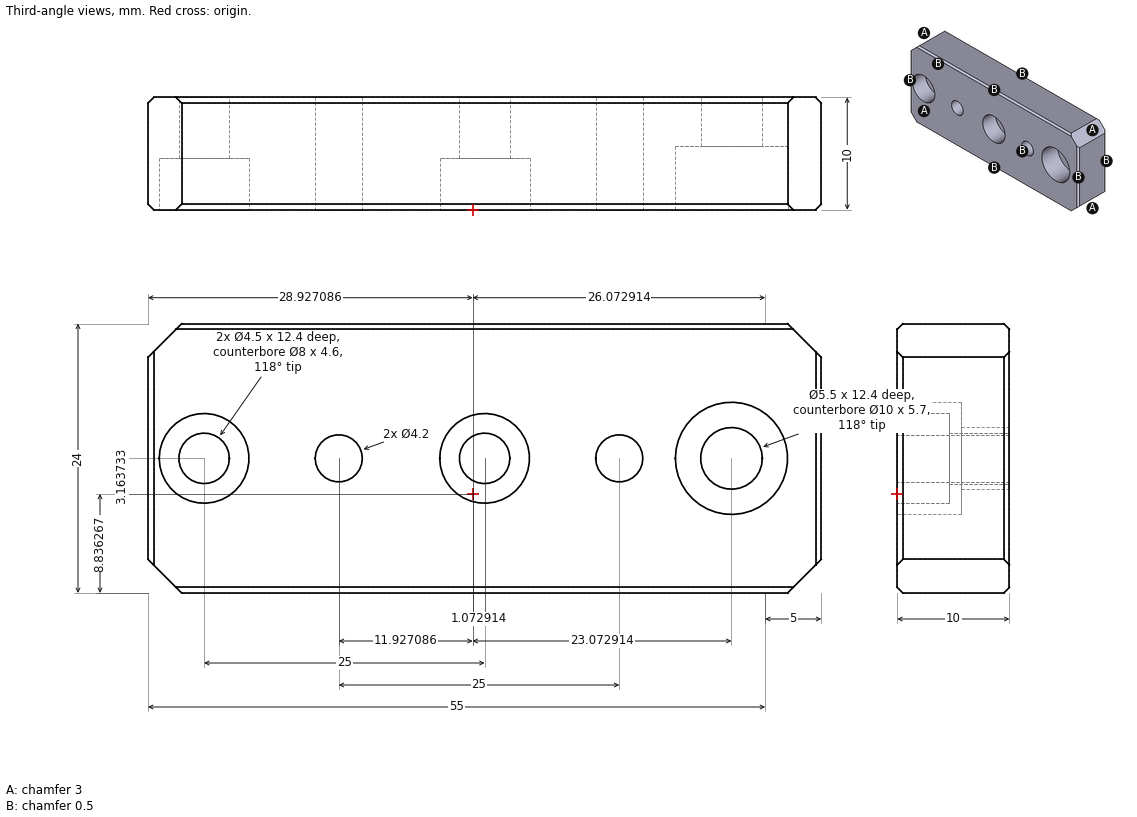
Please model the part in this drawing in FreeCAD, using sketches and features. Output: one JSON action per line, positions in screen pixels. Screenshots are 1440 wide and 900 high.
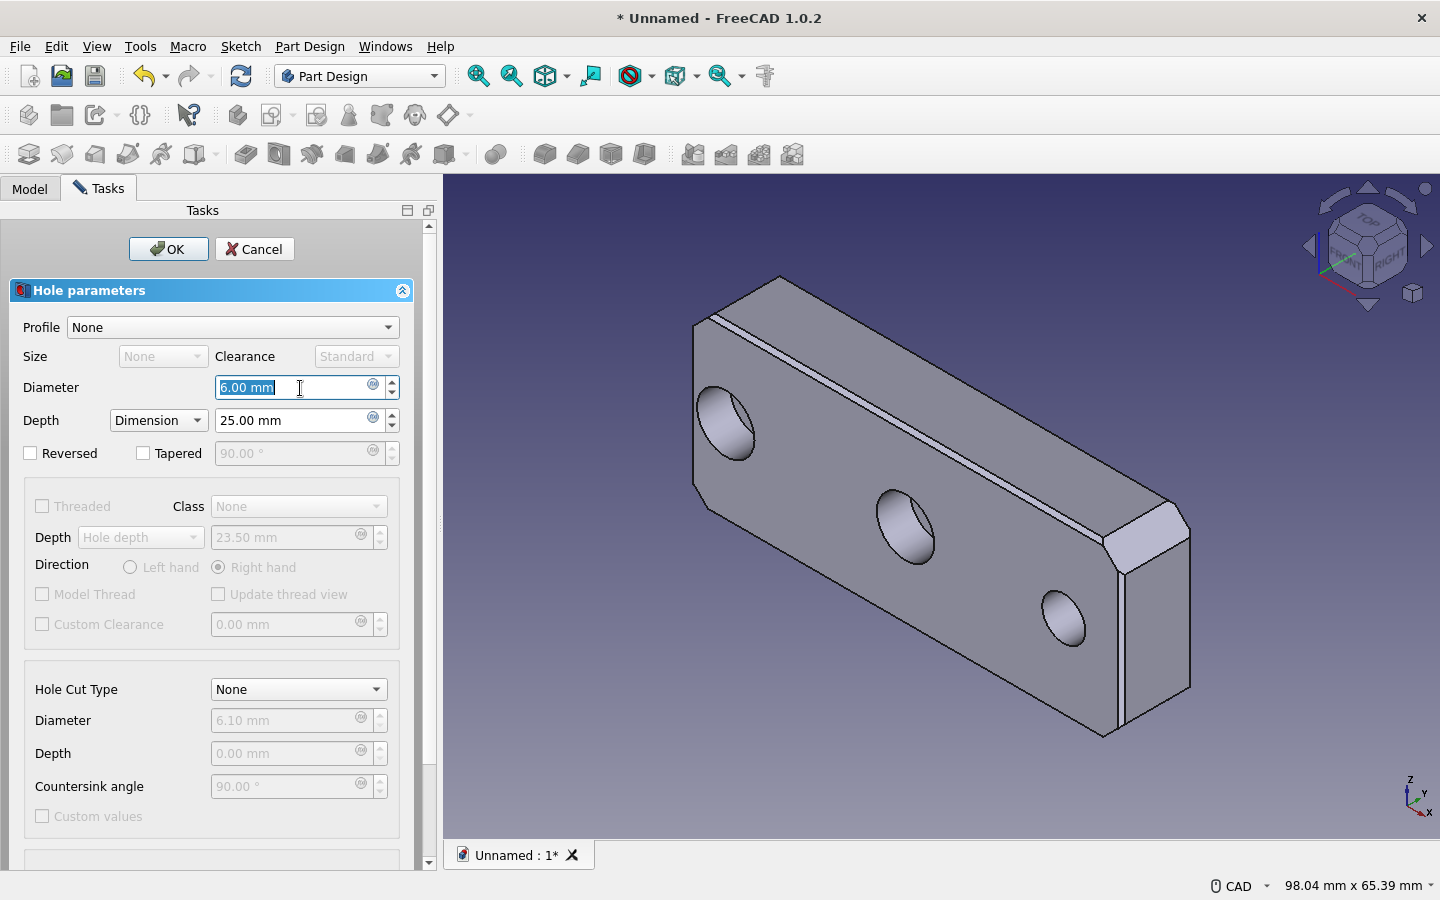
{"action": "type", "text": "5.5"}
{"action": "key", "text": "Tab"}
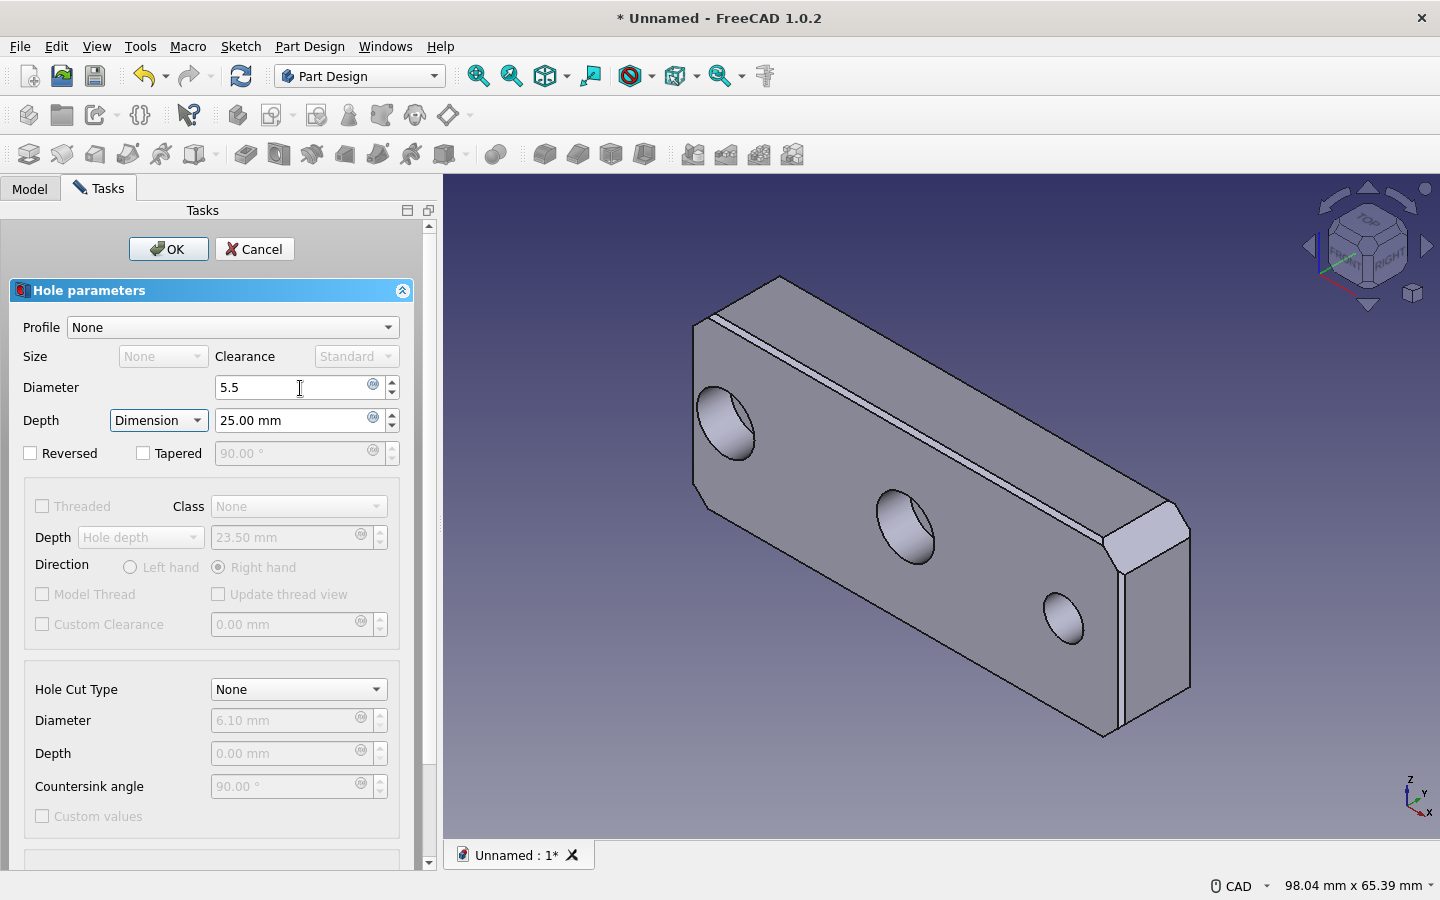
{"action": "triple_click", "coordinate": [300, 420]}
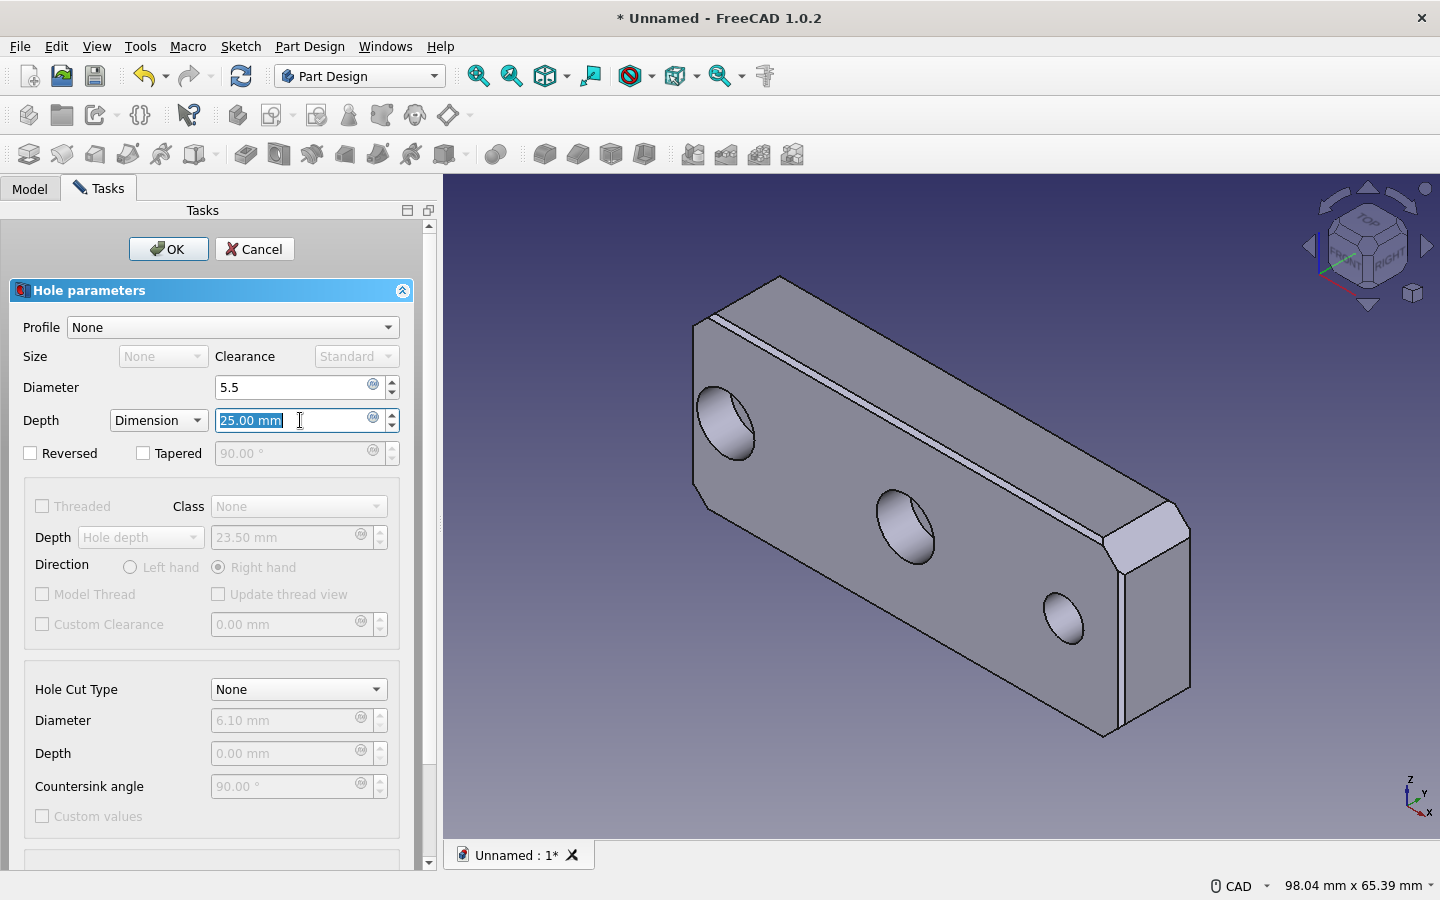
{"action": "type", "text": "12.4"}
{"action": "key", "text": "Tab"}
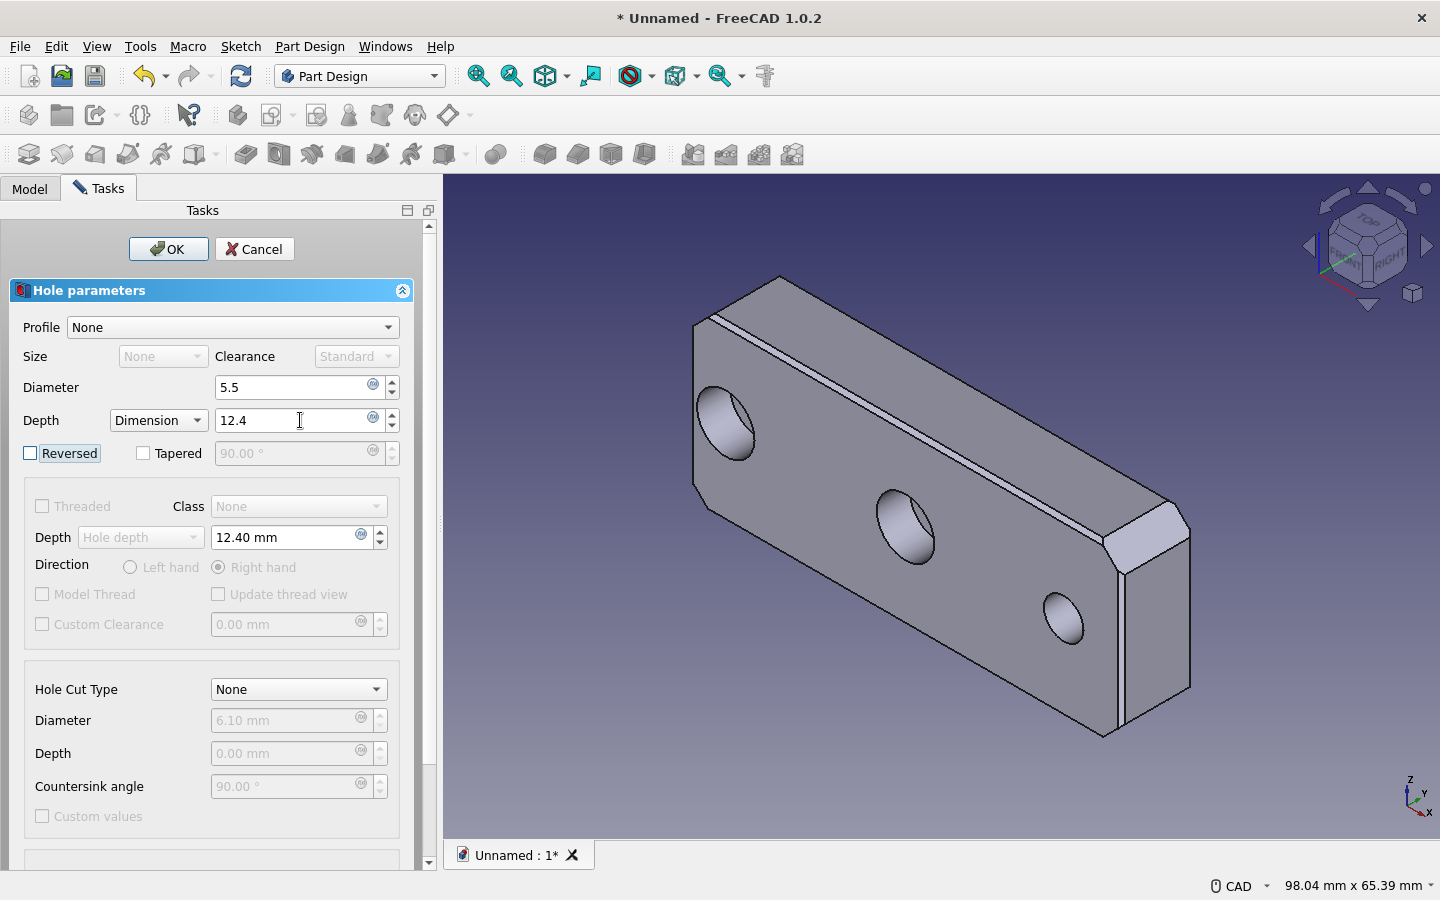
{"action": "left_click", "coordinate": [300, 690]}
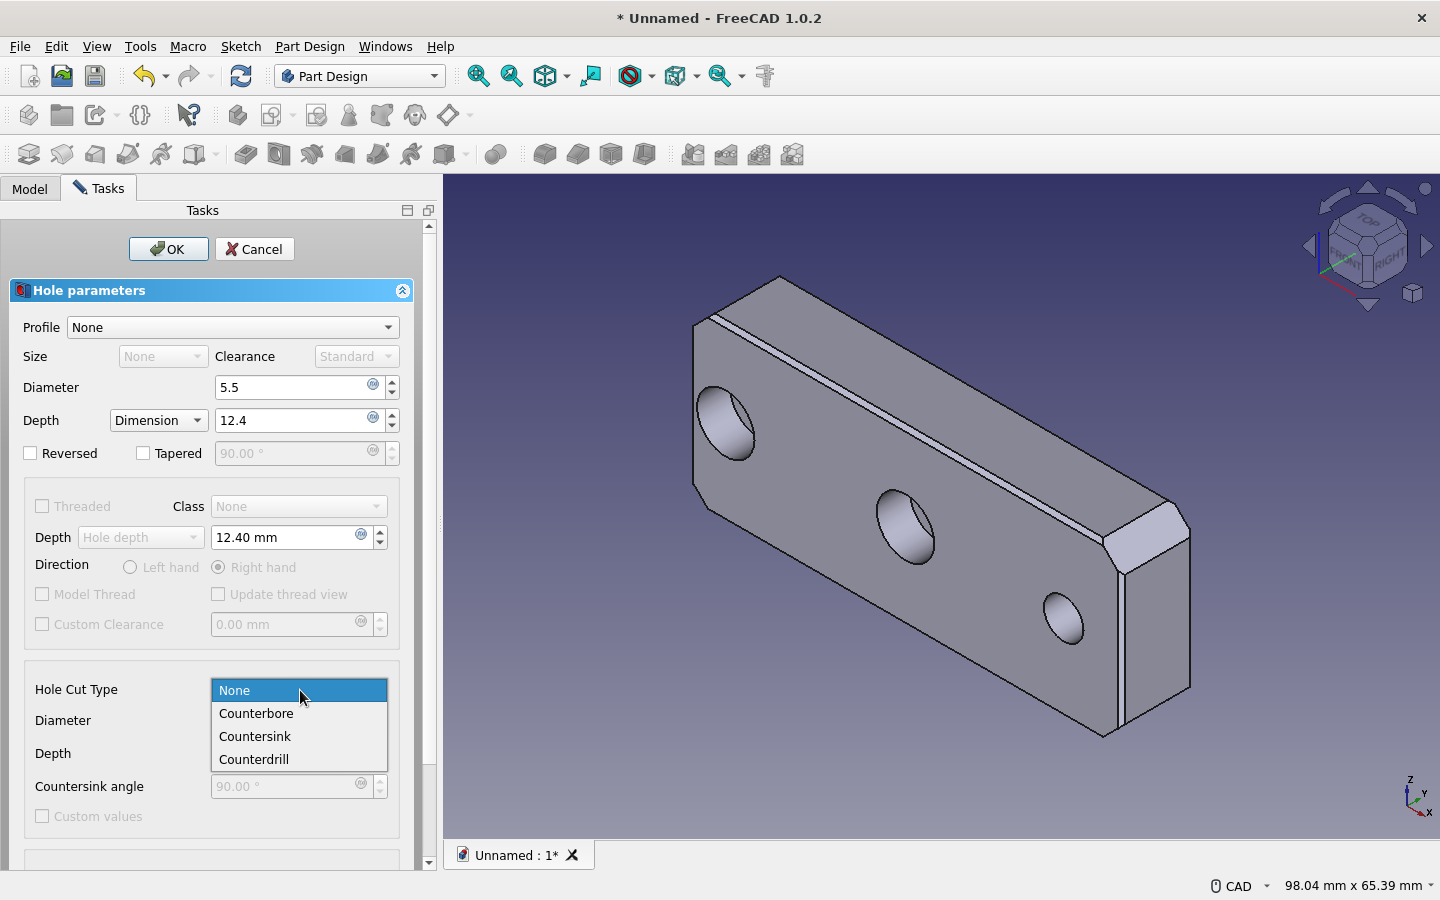
{"action": "left_click", "coordinate": [298, 714]}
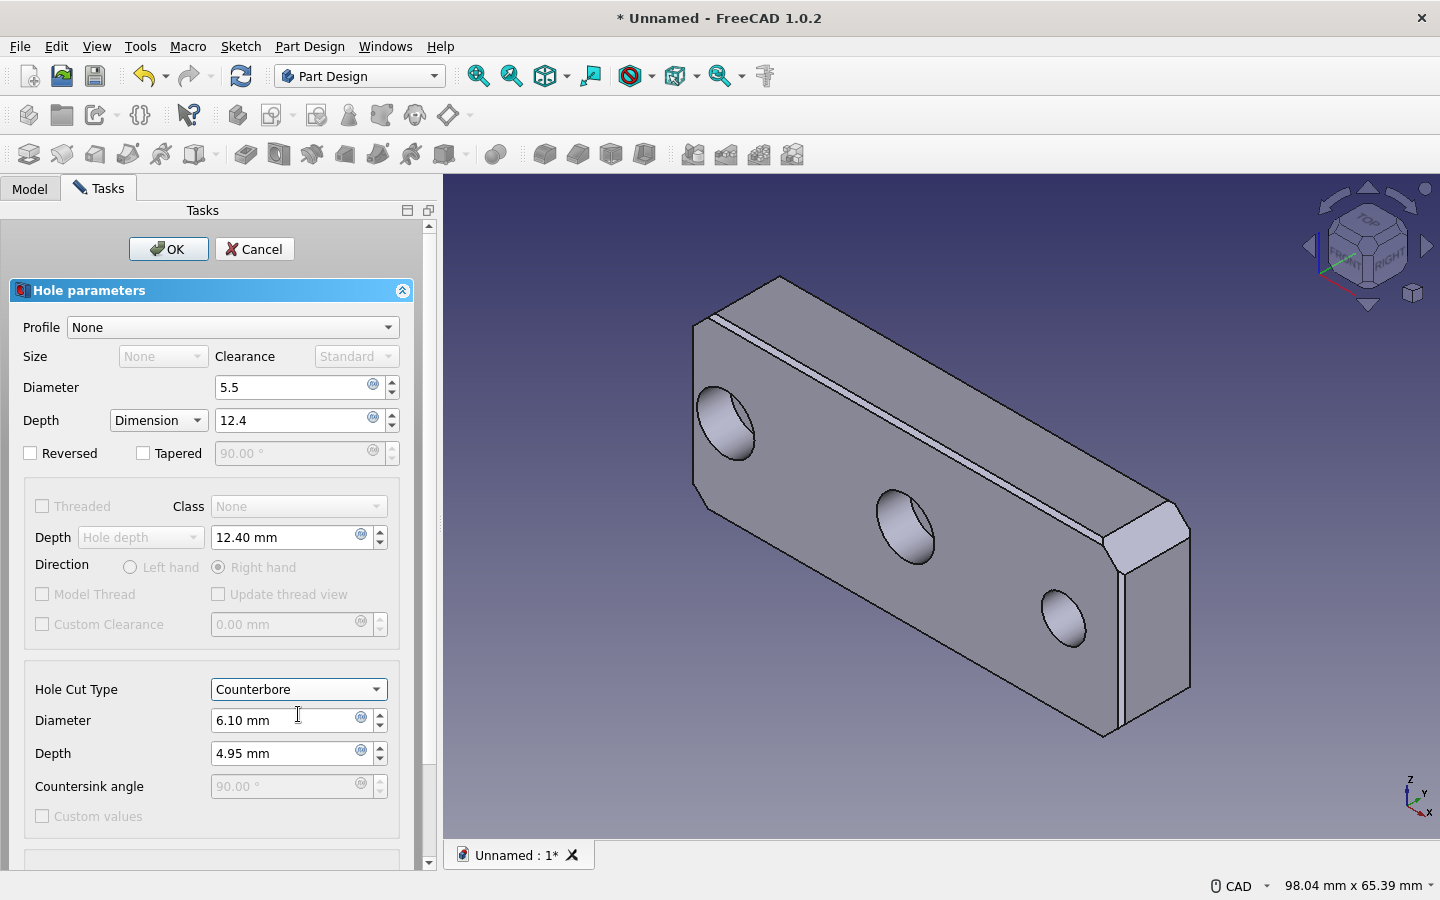
{"action": "triple_click", "coordinate": [292, 720]}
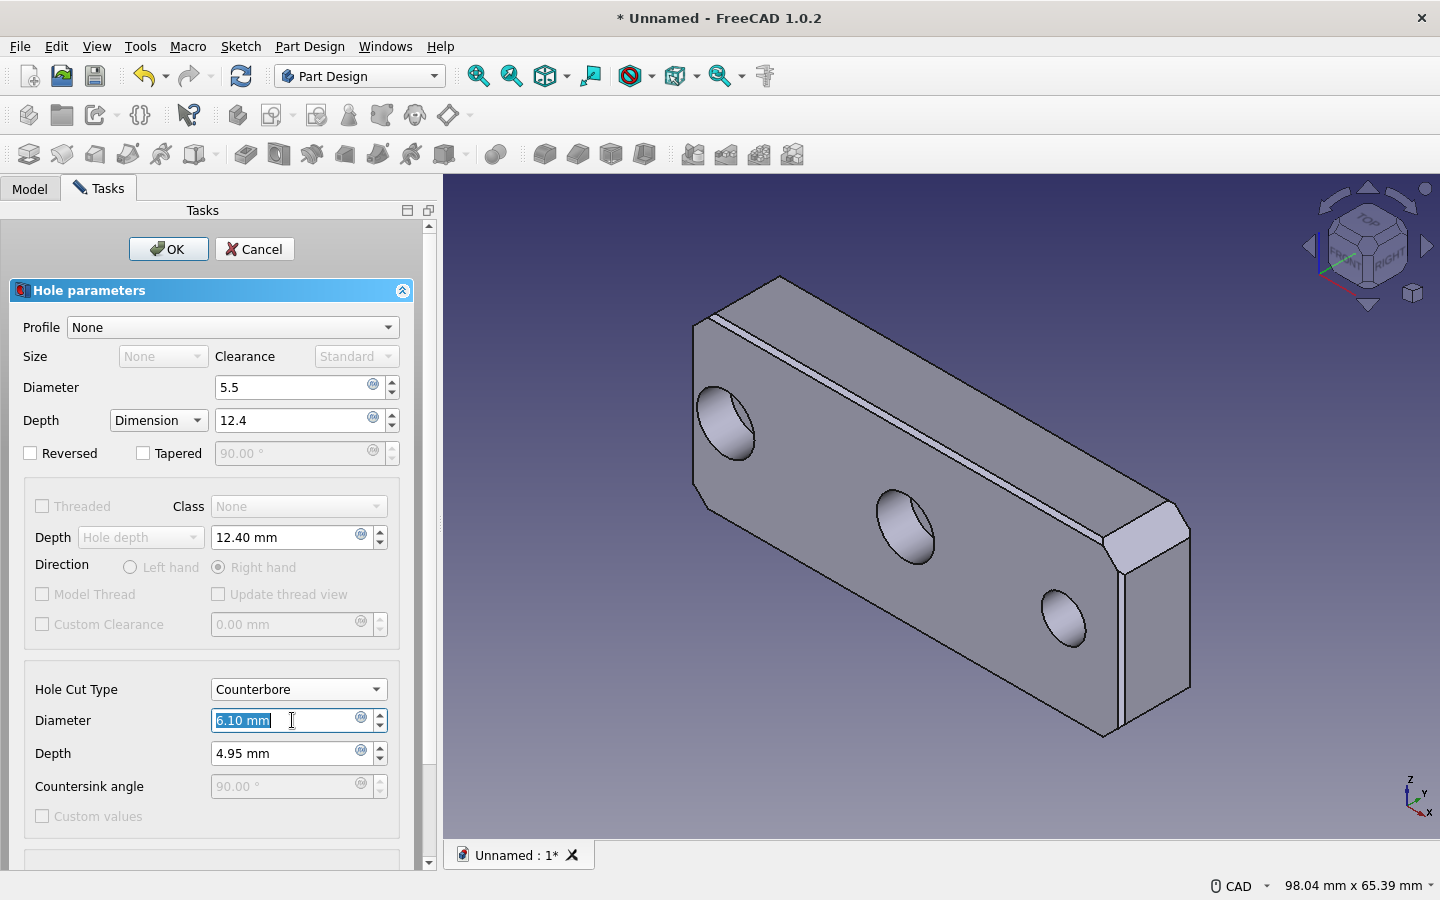
{"action": "type", "text": "10"}
{"action": "key", "text": "Tab"}